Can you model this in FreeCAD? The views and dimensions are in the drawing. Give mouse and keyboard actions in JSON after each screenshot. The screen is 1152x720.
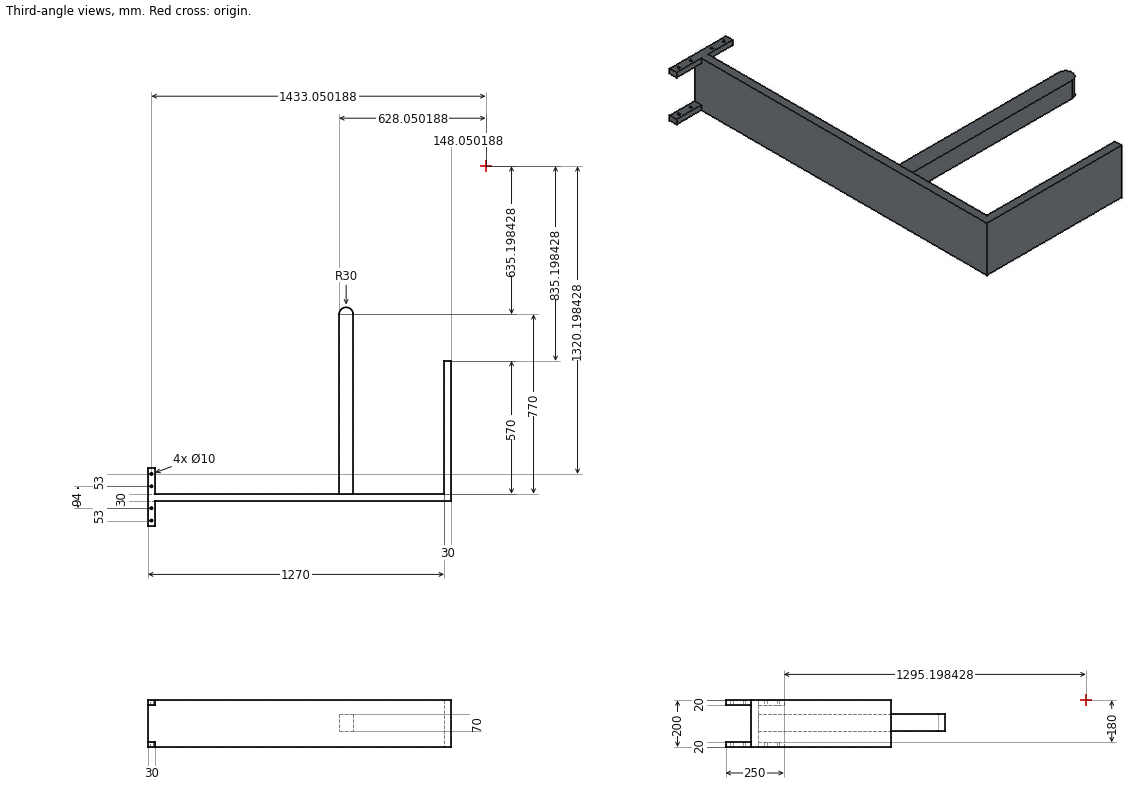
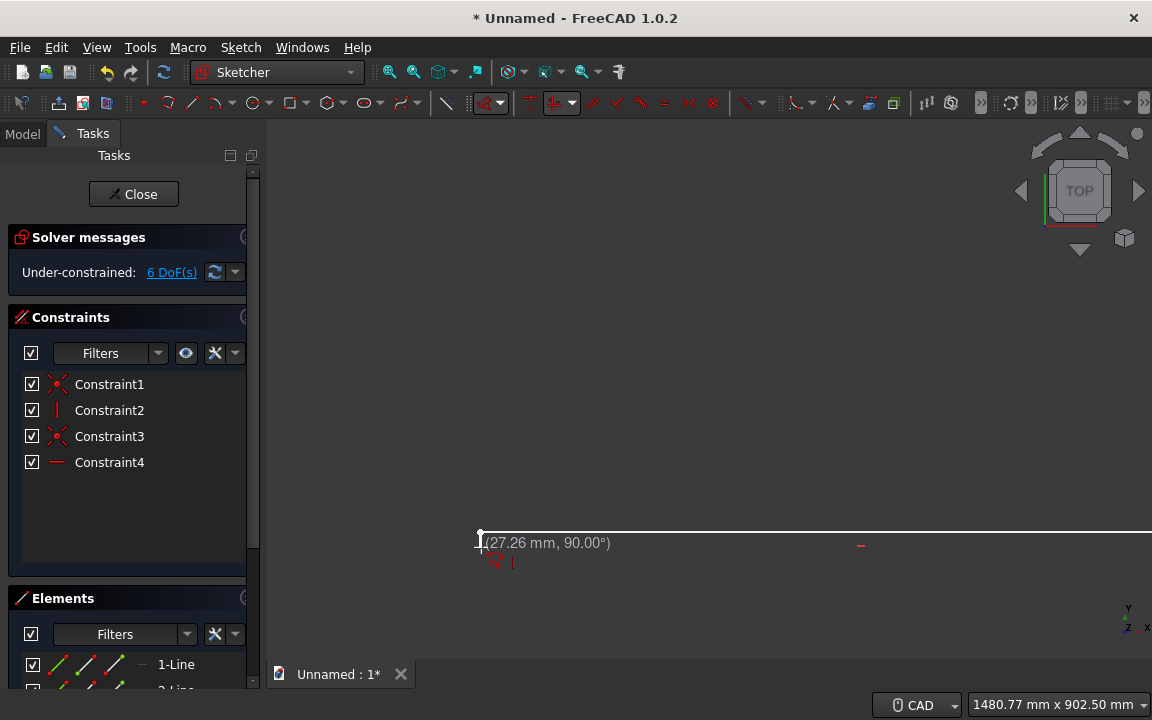
{"action": "left_click", "coordinate": [481, 546]}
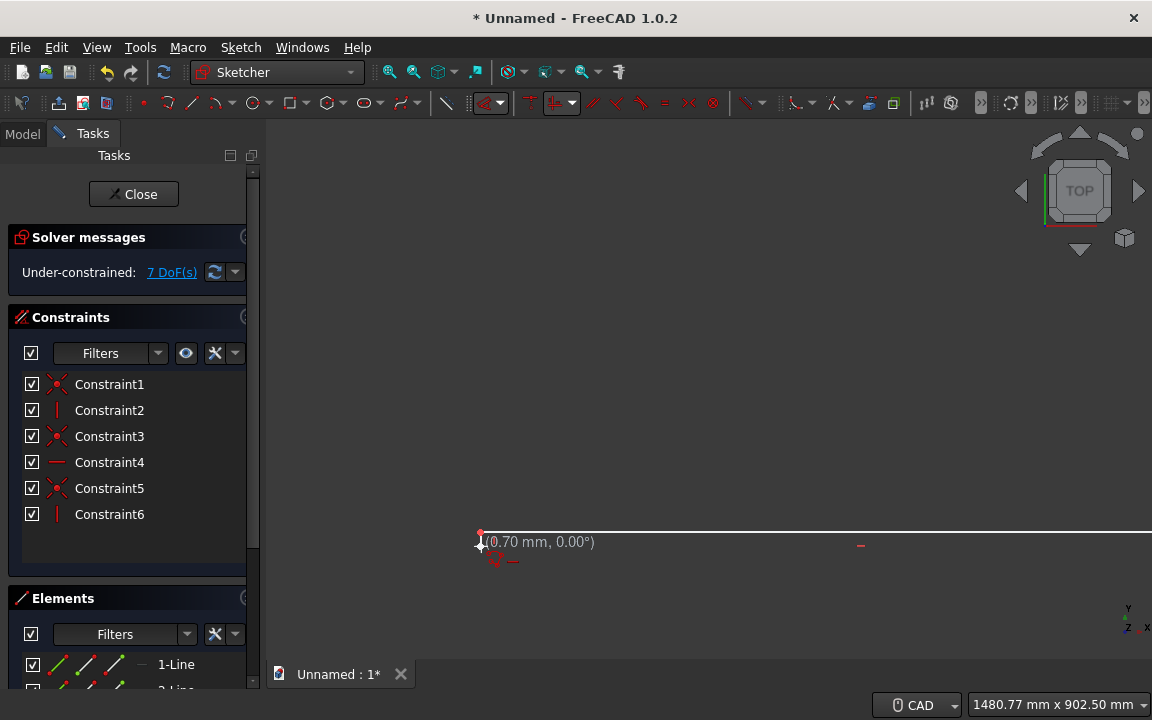
{"action": "scroll", "coordinate": [481, 547], "scroll_direction": "down", "scroll_amount": 5}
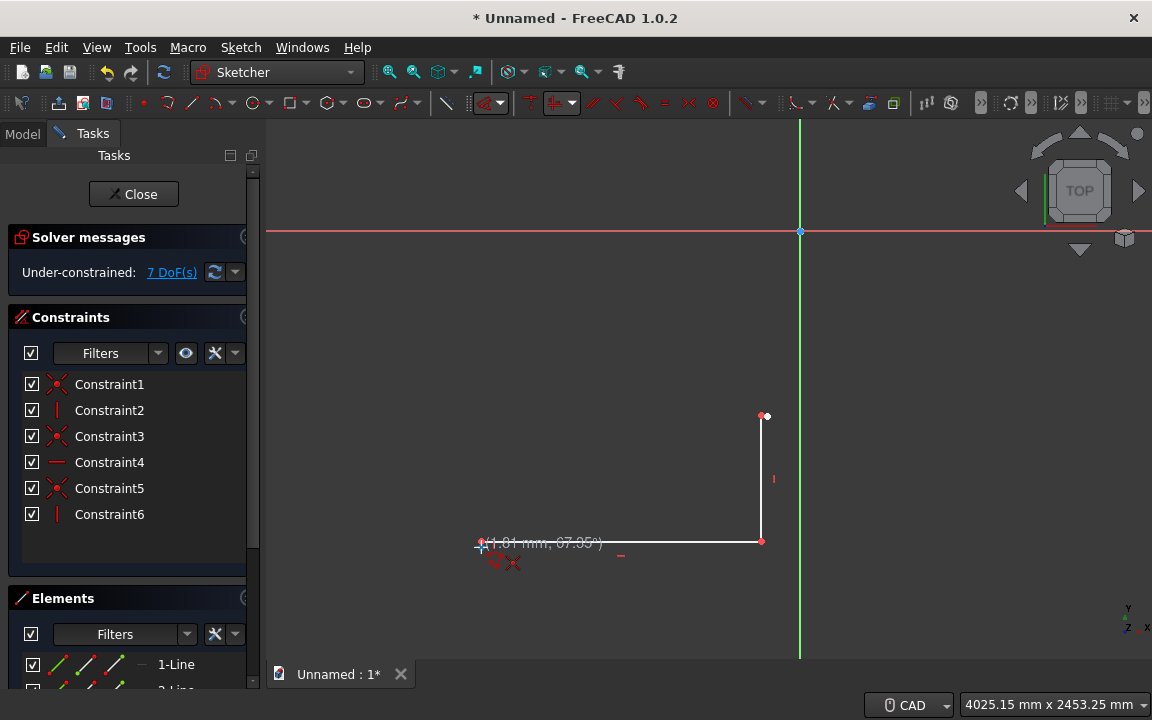
{"action": "scroll", "coordinate": [768, 547], "scroll_direction": "up", "scroll_amount": 3}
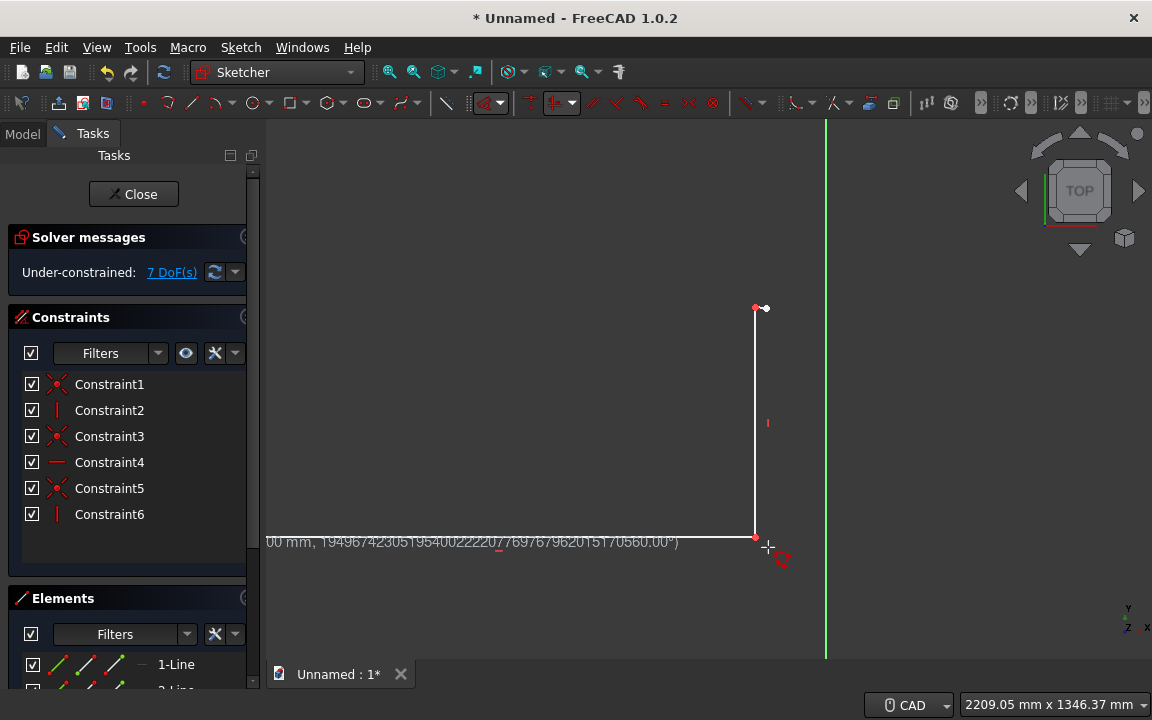
{"action": "left_click", "coordinate": [767, 547]}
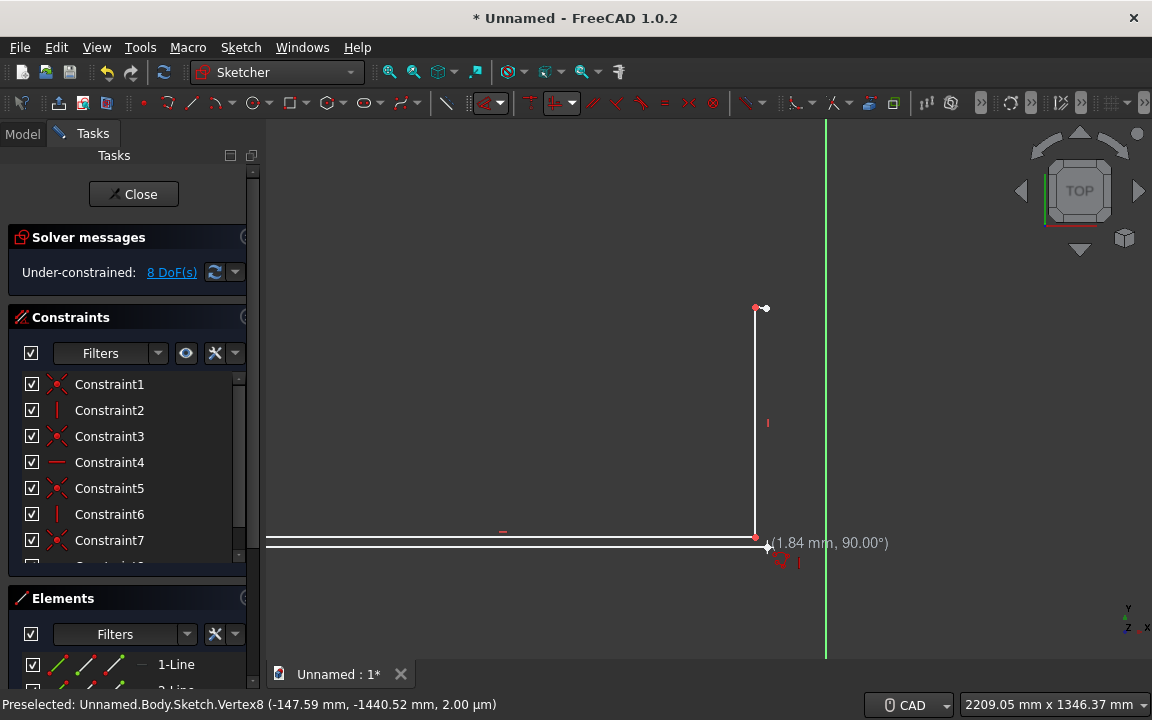
{"action": "scroll", "coordinate": [767, 306], "scroll_direction": "up", "scroll_amount": 5}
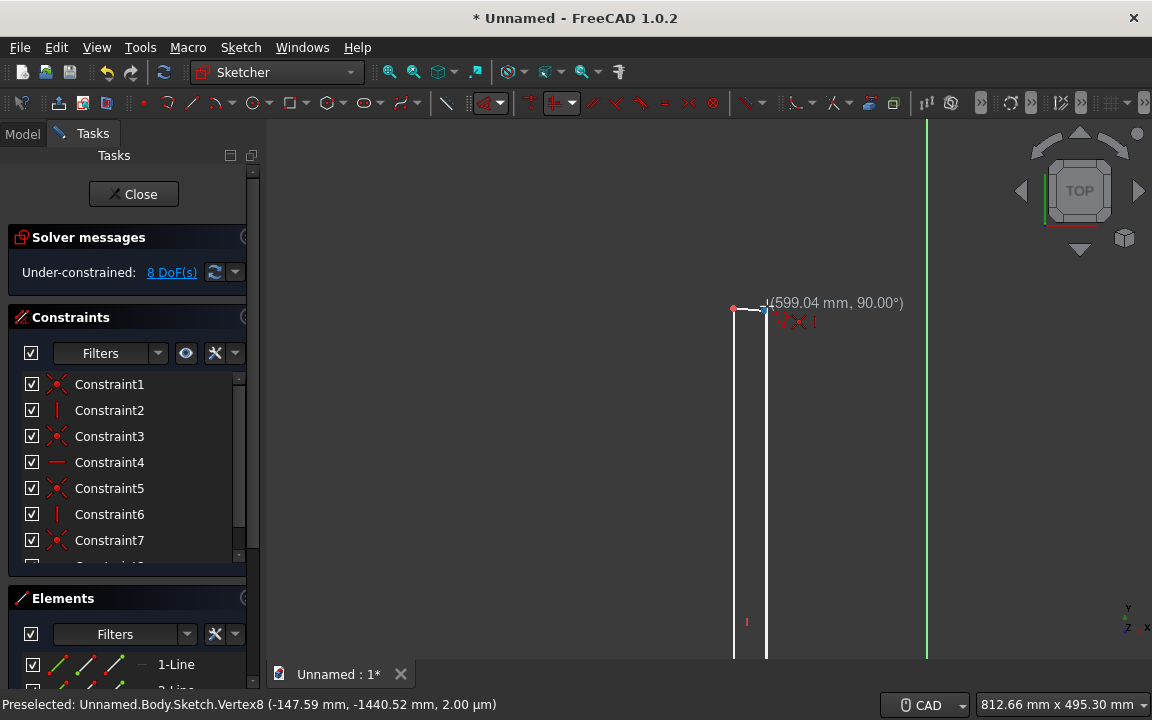
{"action": "left_click", "coordinate": [765, 311]}
{"action": "key", "text": "Escape"}
{"action": "key", "text": "Escape"}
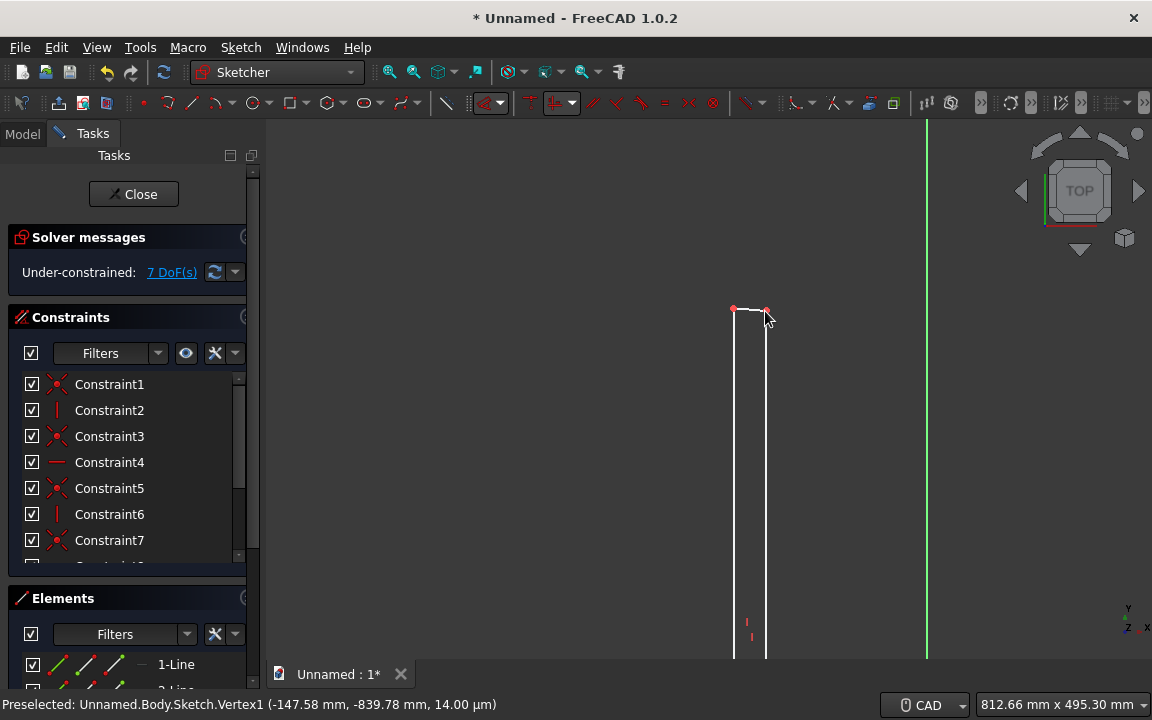
{"action": "scroll", "coordinate": [756, 310], "scroll_direction": "up", "scroll_amount": 2}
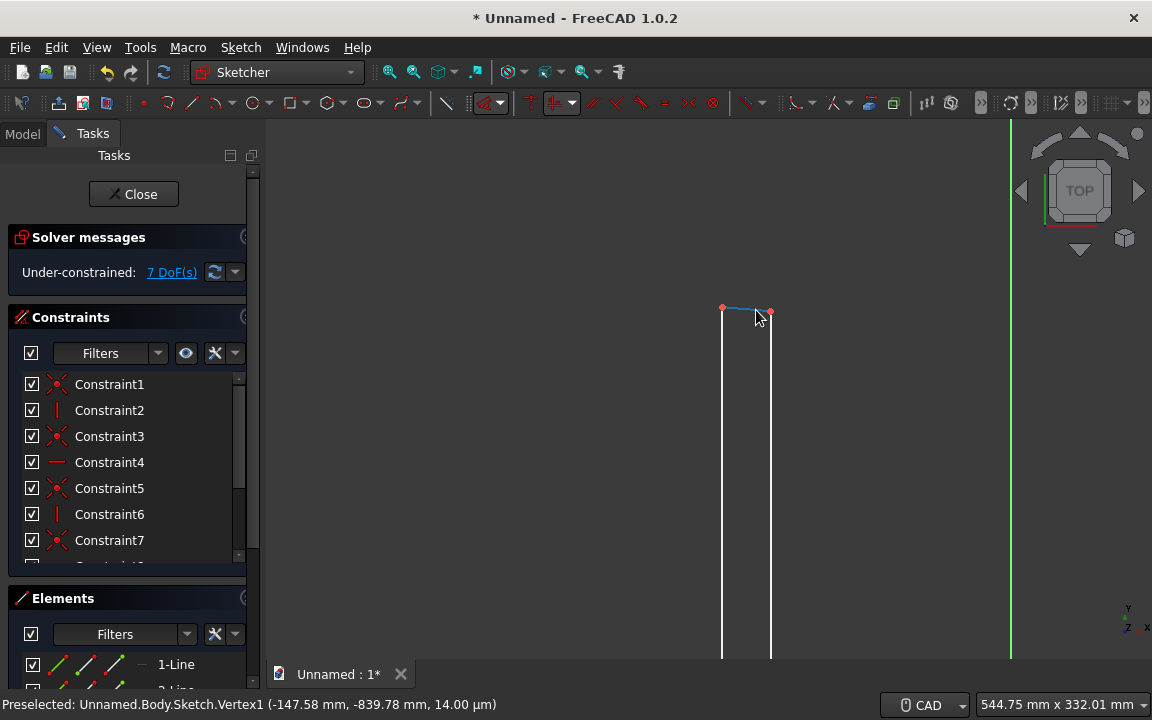
{"action": "left_click", "coordinate": [756, 310]}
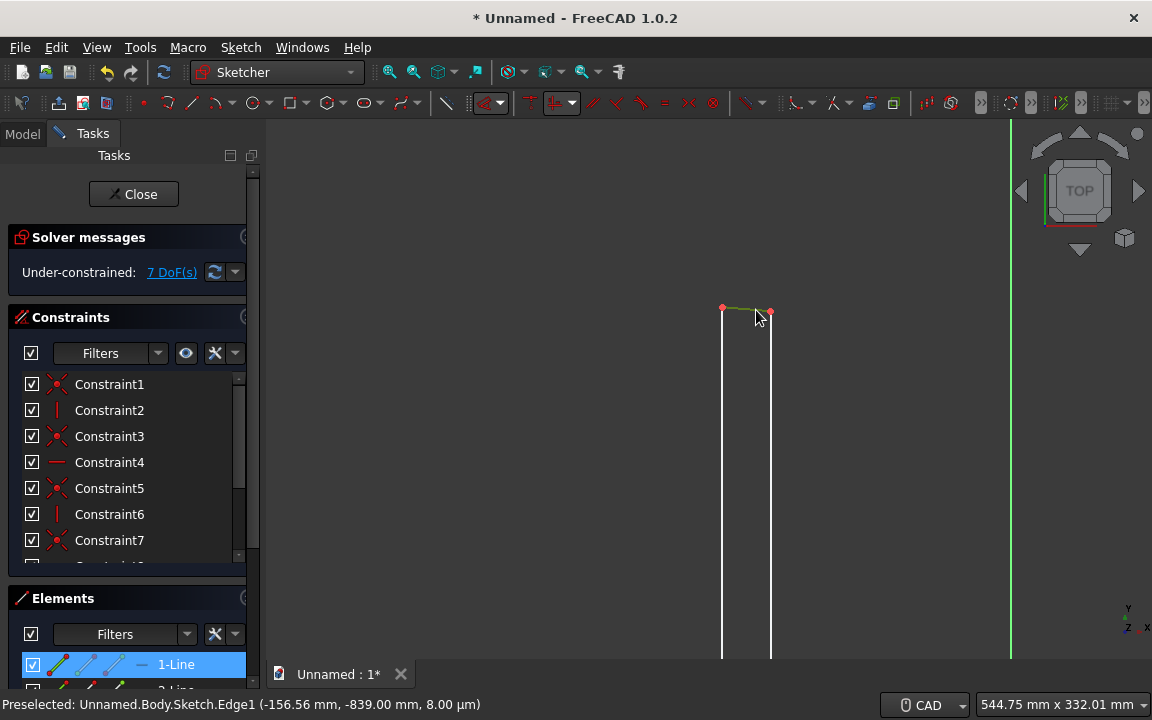
{"action": "key", "text": "h"}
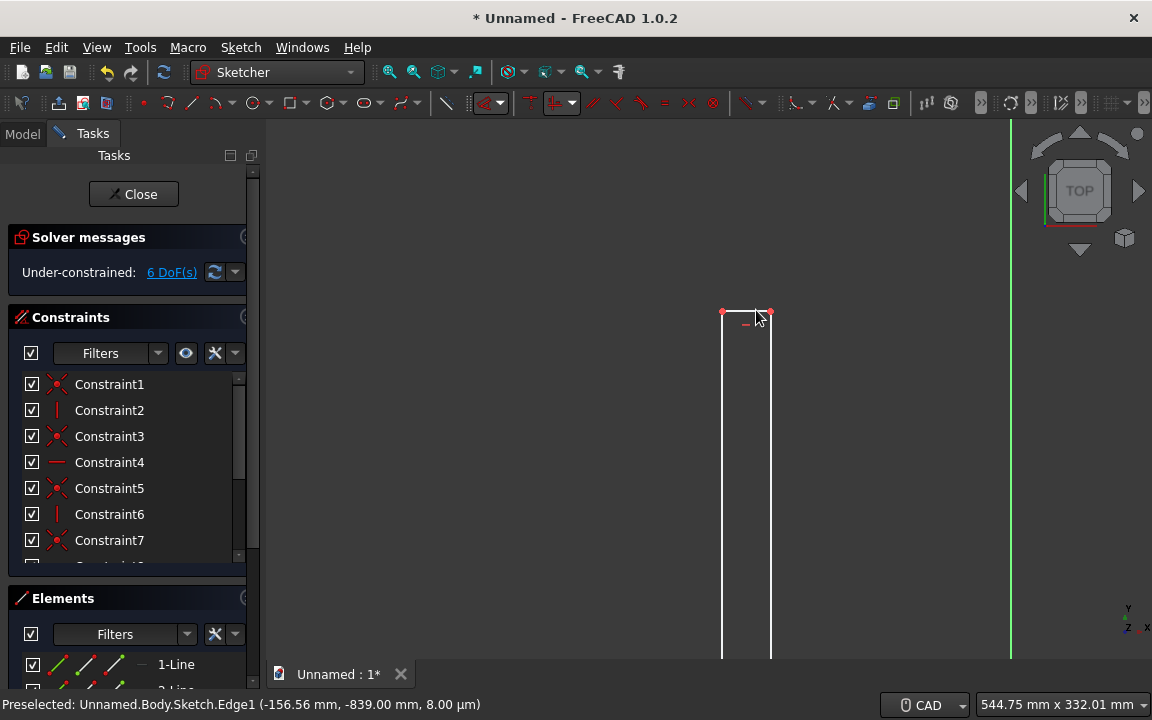
{"action": "left_click", "coordinate": [756, 311]}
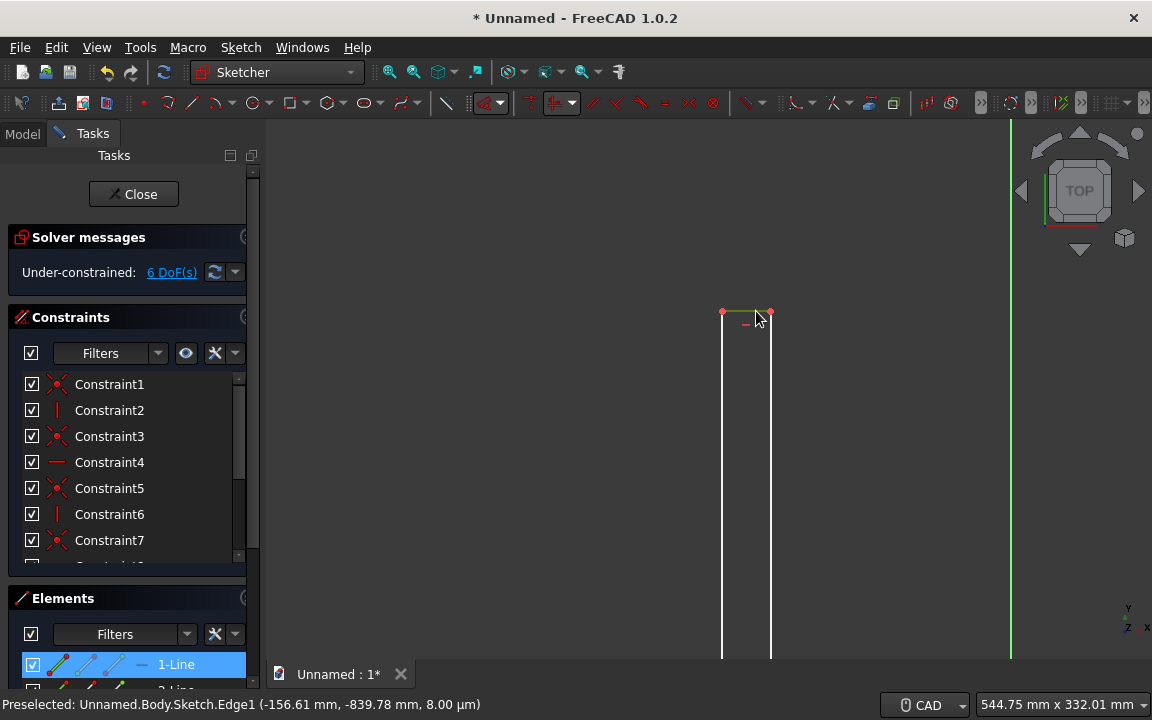
{"action": "left_click", "coordinate": [502, 104]}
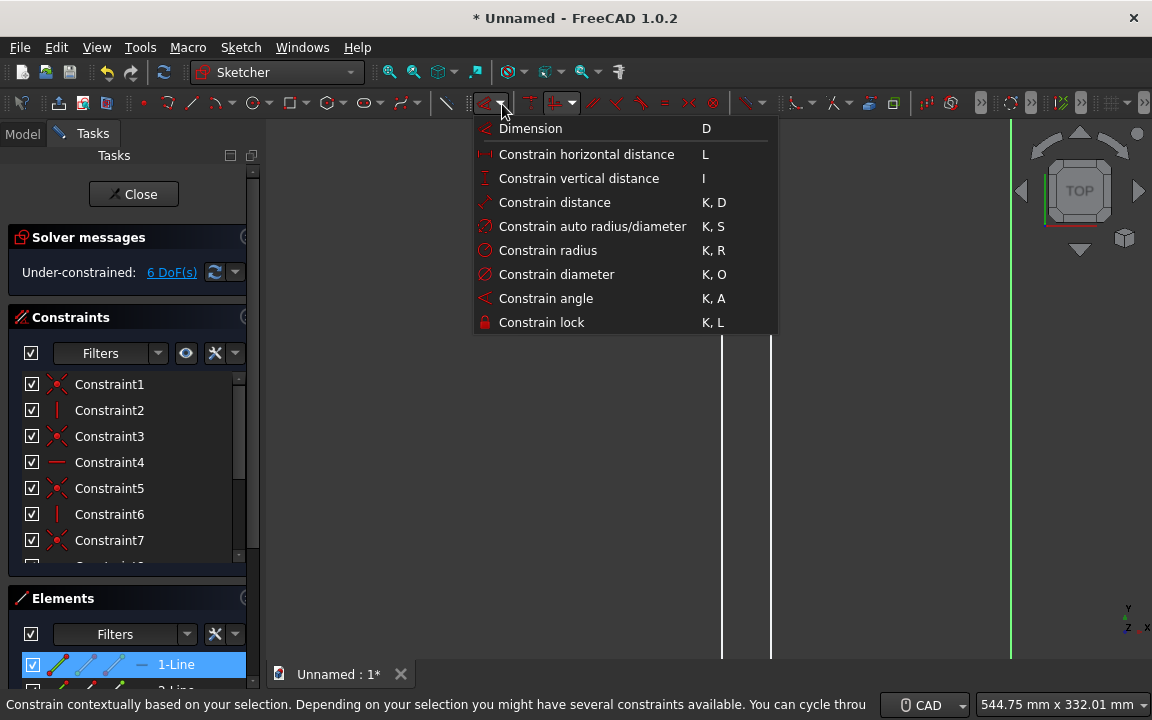
{"action": "left_click", "coordinate": [626, 154]}